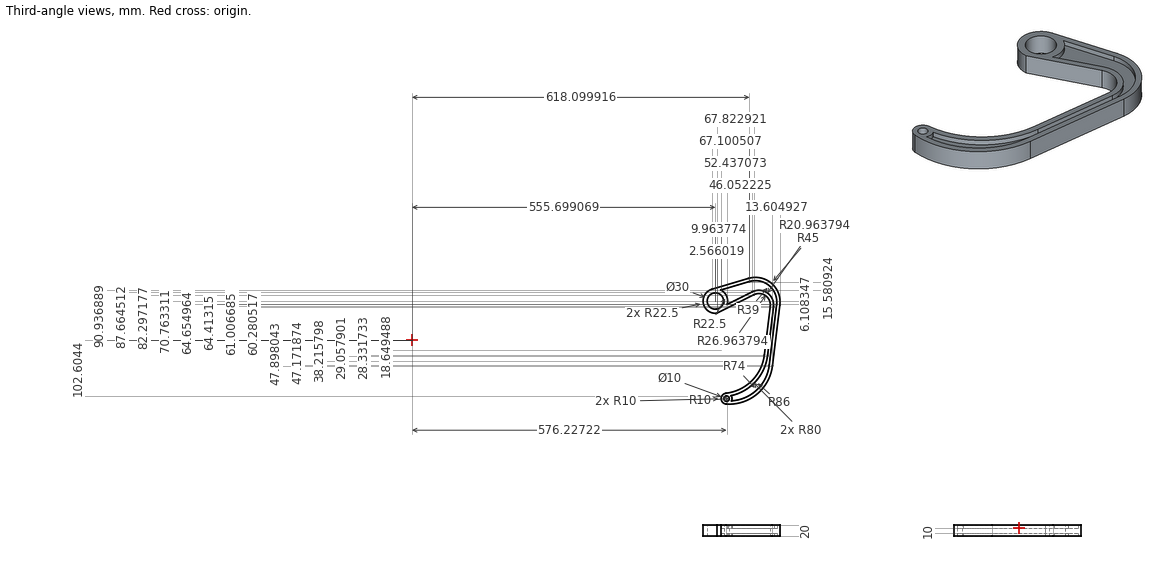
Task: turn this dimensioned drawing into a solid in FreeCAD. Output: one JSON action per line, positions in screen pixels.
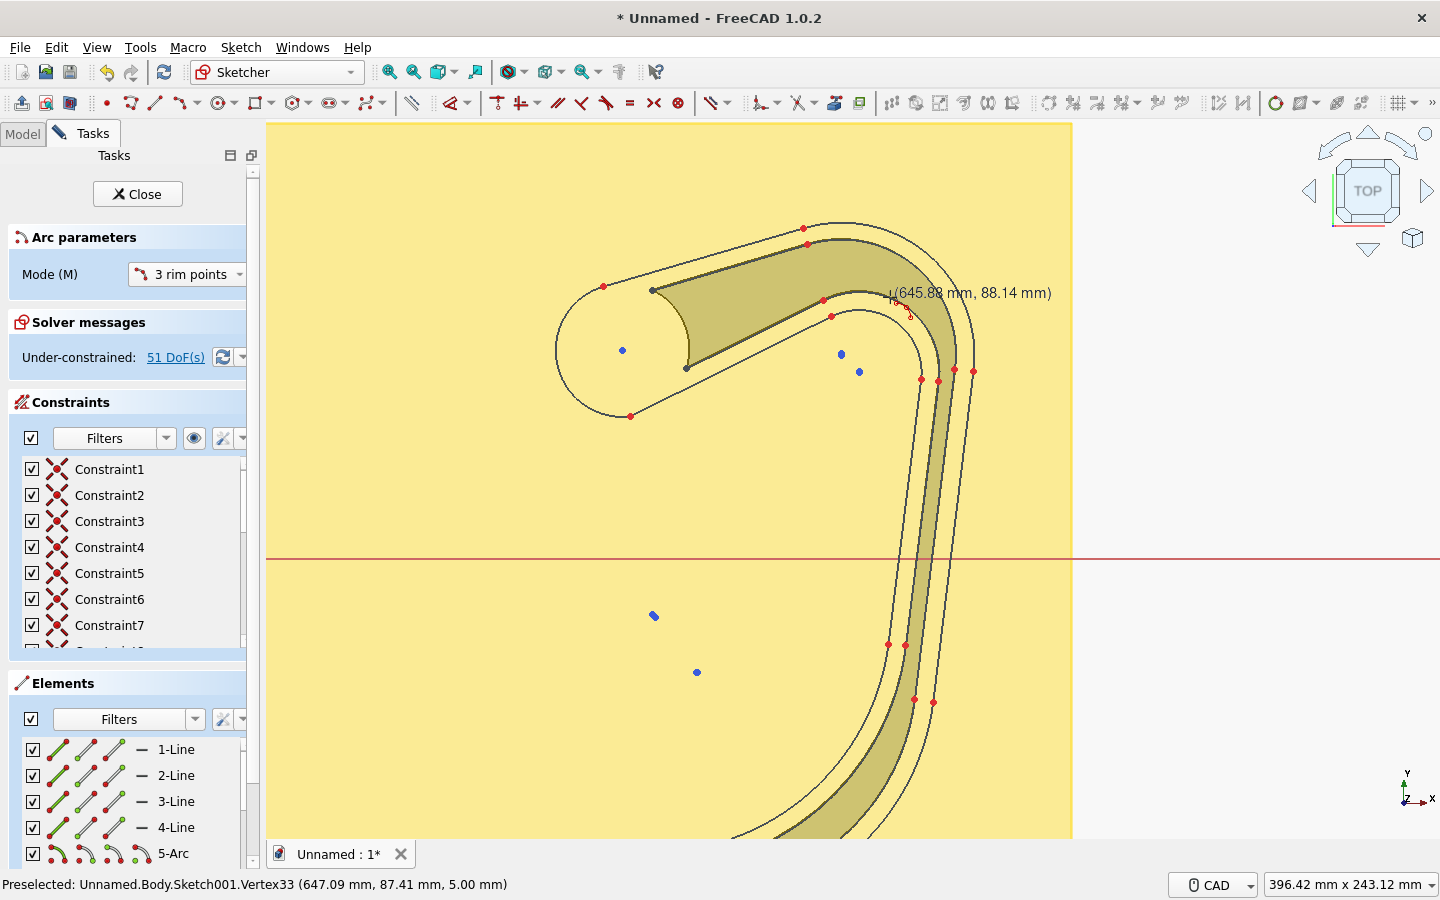
{"action": "left_click", "coordinate": [687, 369]}
{"action": "left_click", "coordinate": [653, 291]}
{"action": "left_click", "coordinate": [684, 322]}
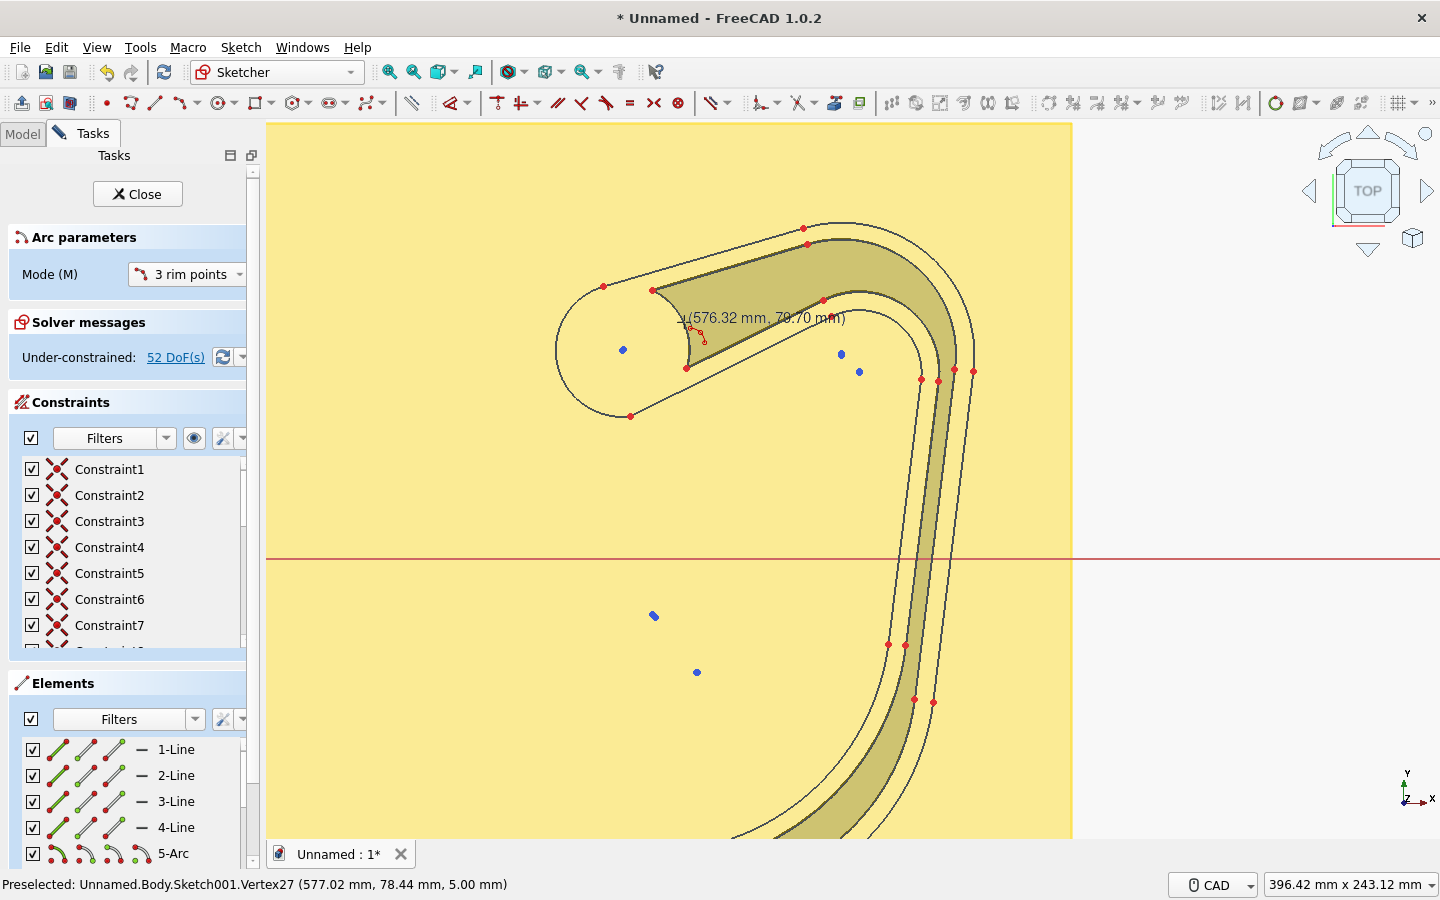
{"action": "left_click", "coordinate": [218, 104]}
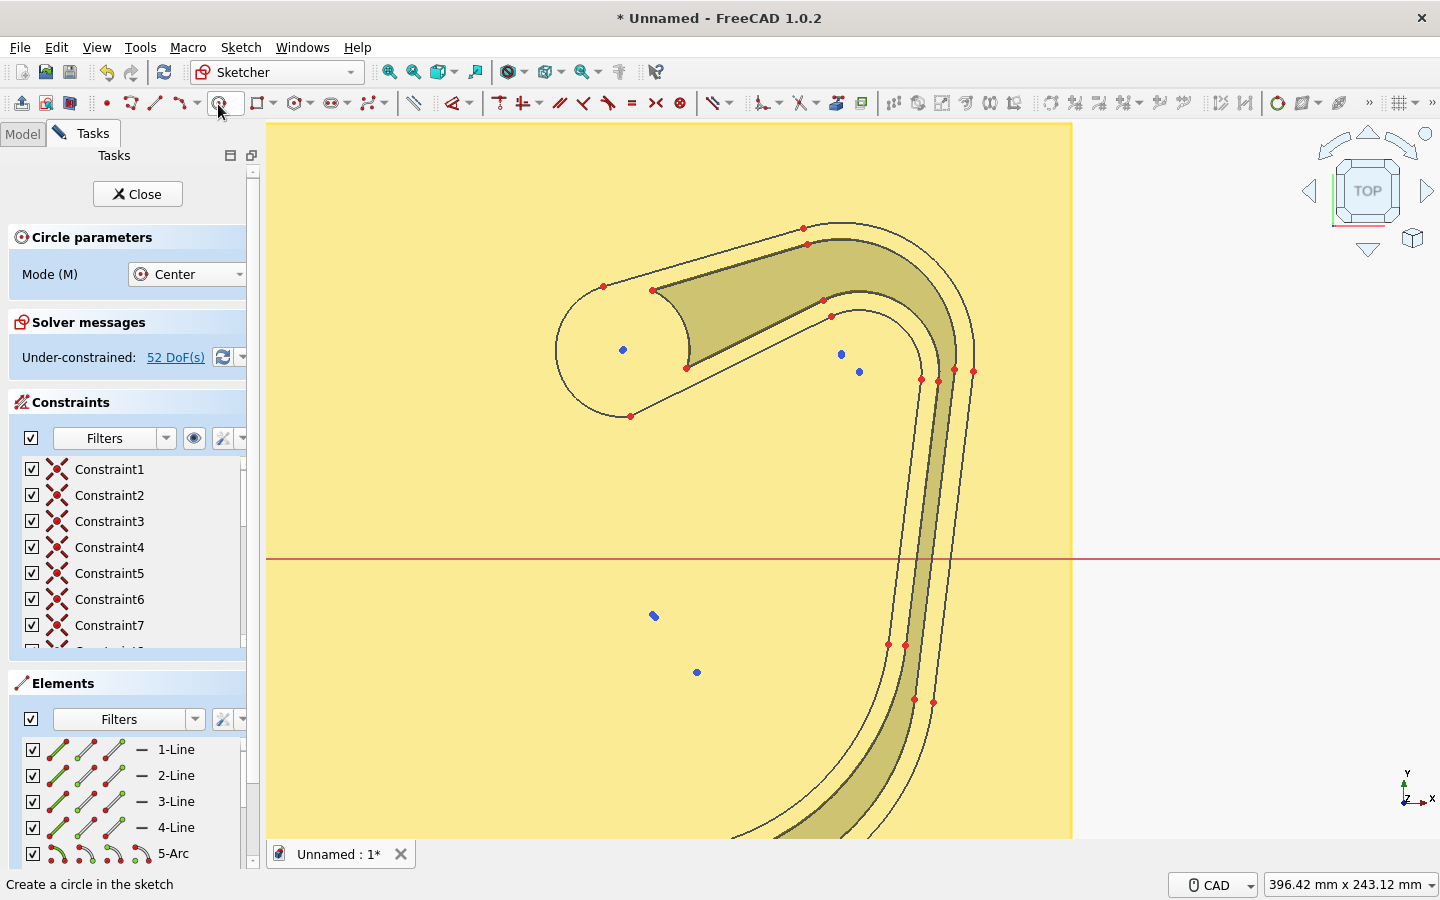
{"action": "scroll", "coordinate": [824, 299], "scroll_direction": "down", "scroll_amount": 2}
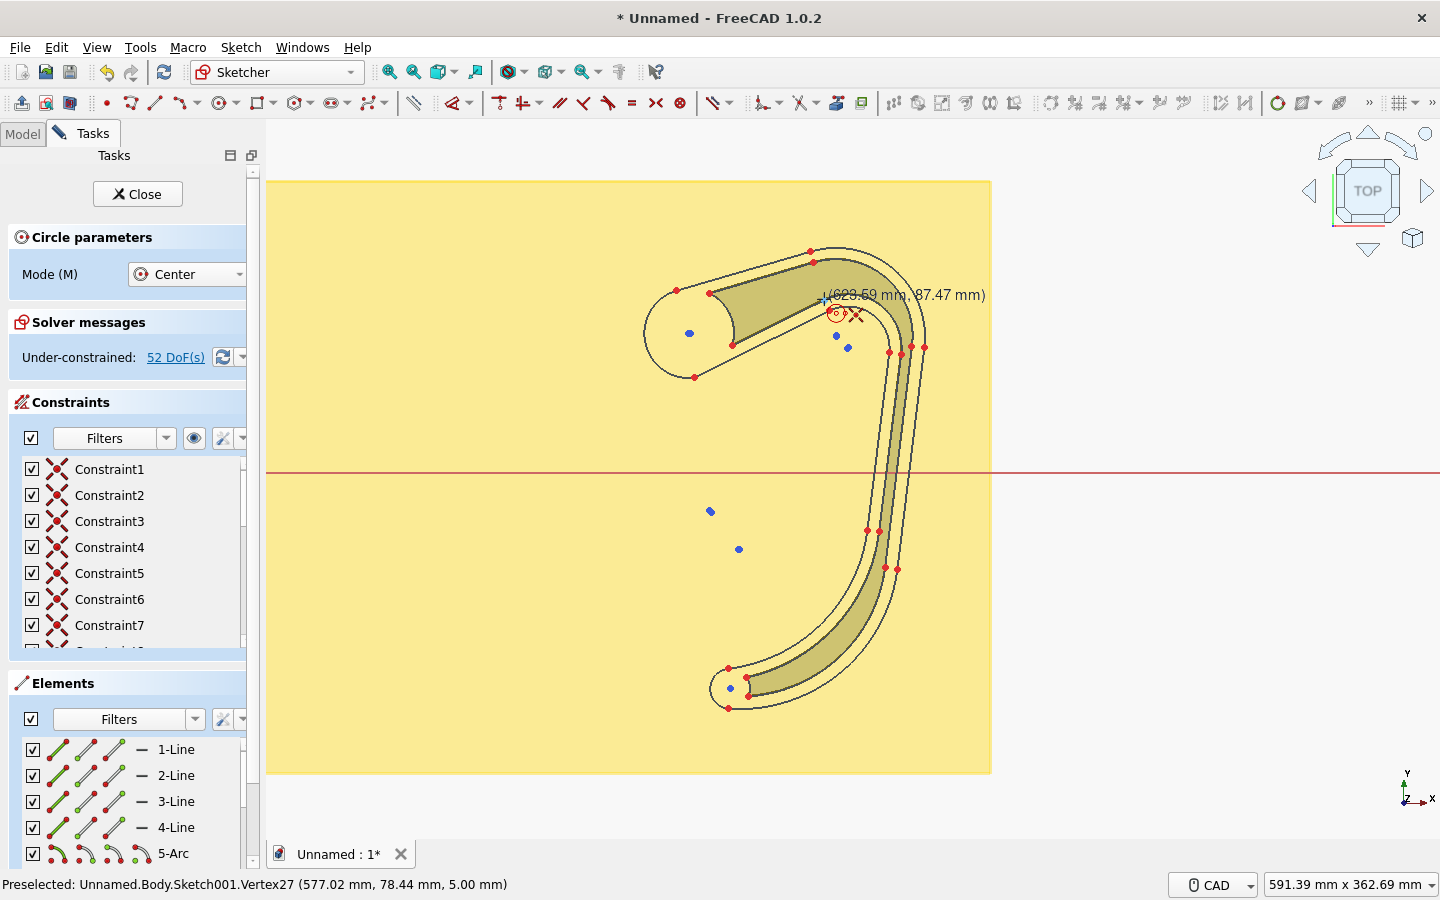
{"action": "scroll", "coordinate": [730, 688], "scroll_direction": "up", "scroll_amount": 5}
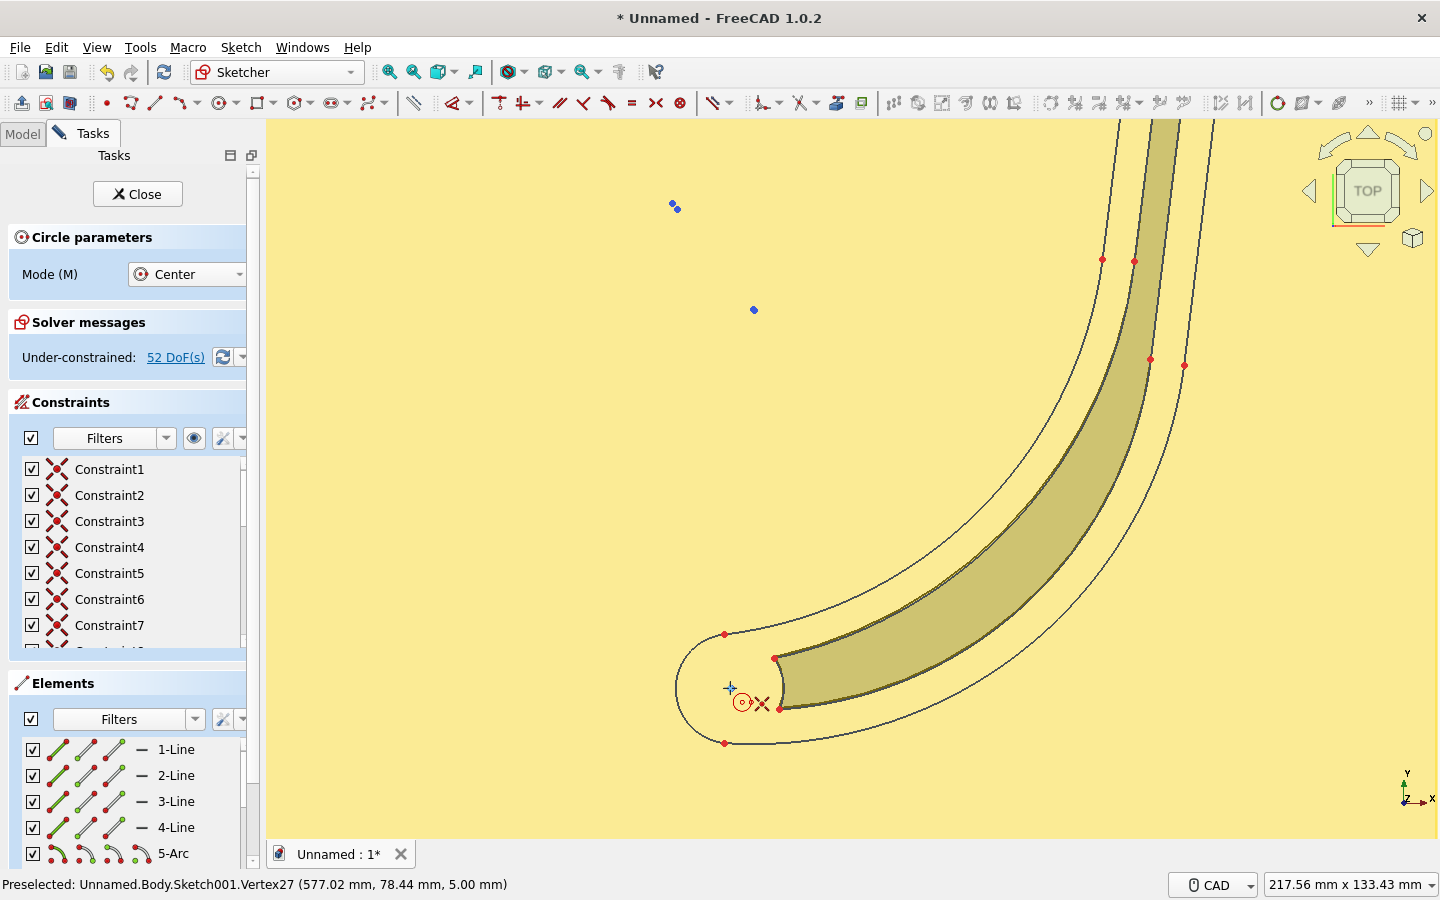
{"action": "left_click", "coordinate": [730, 686]}
{"action": "mouse_move", "coordinate": [749, 667]}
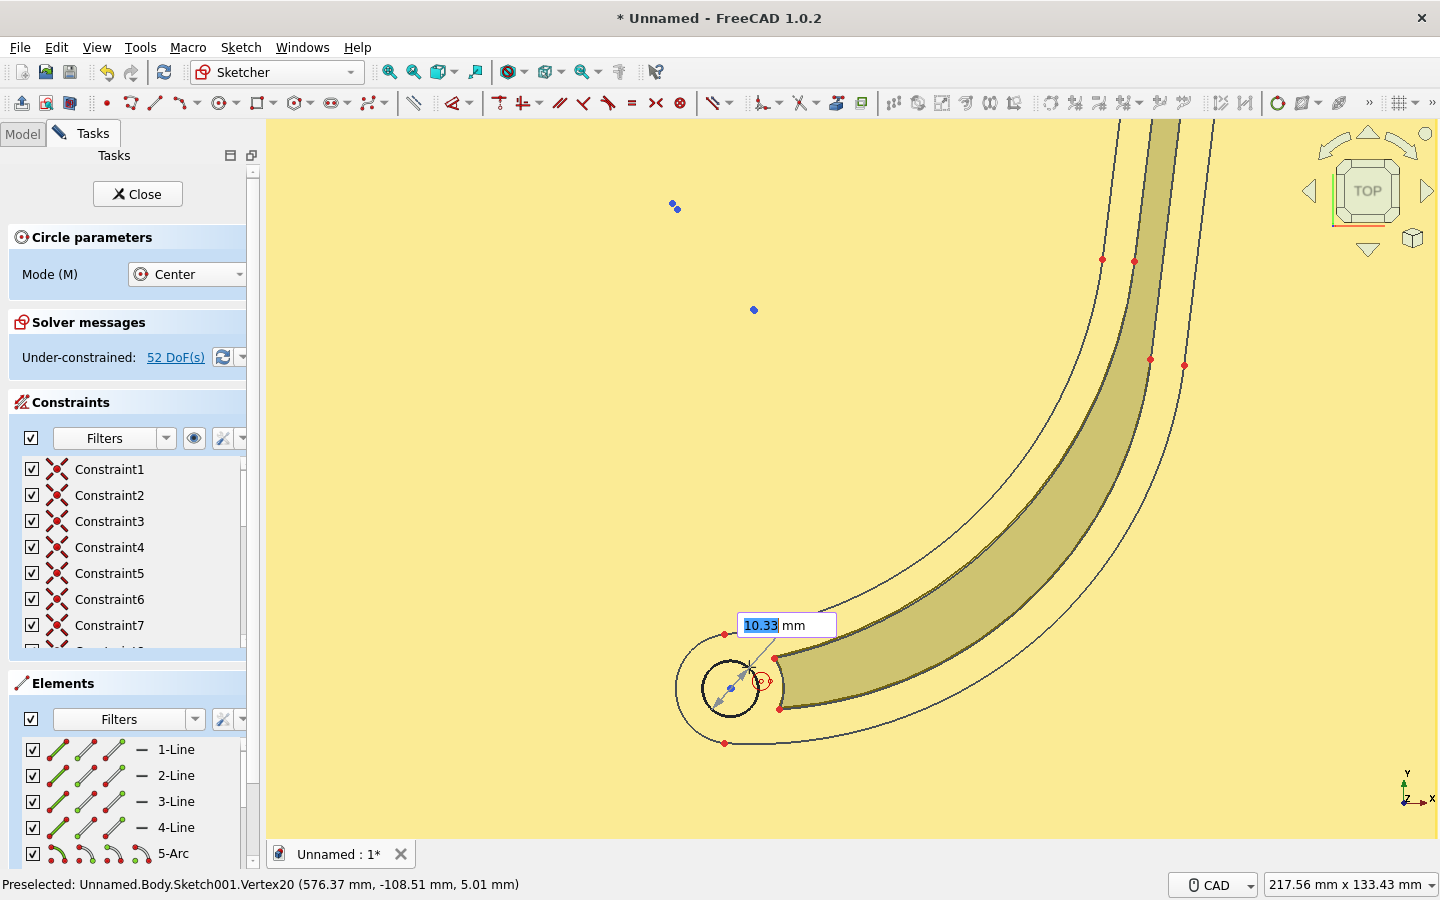
{"action": "type", "text": "10"}
{"action": "key", "text": "Return"}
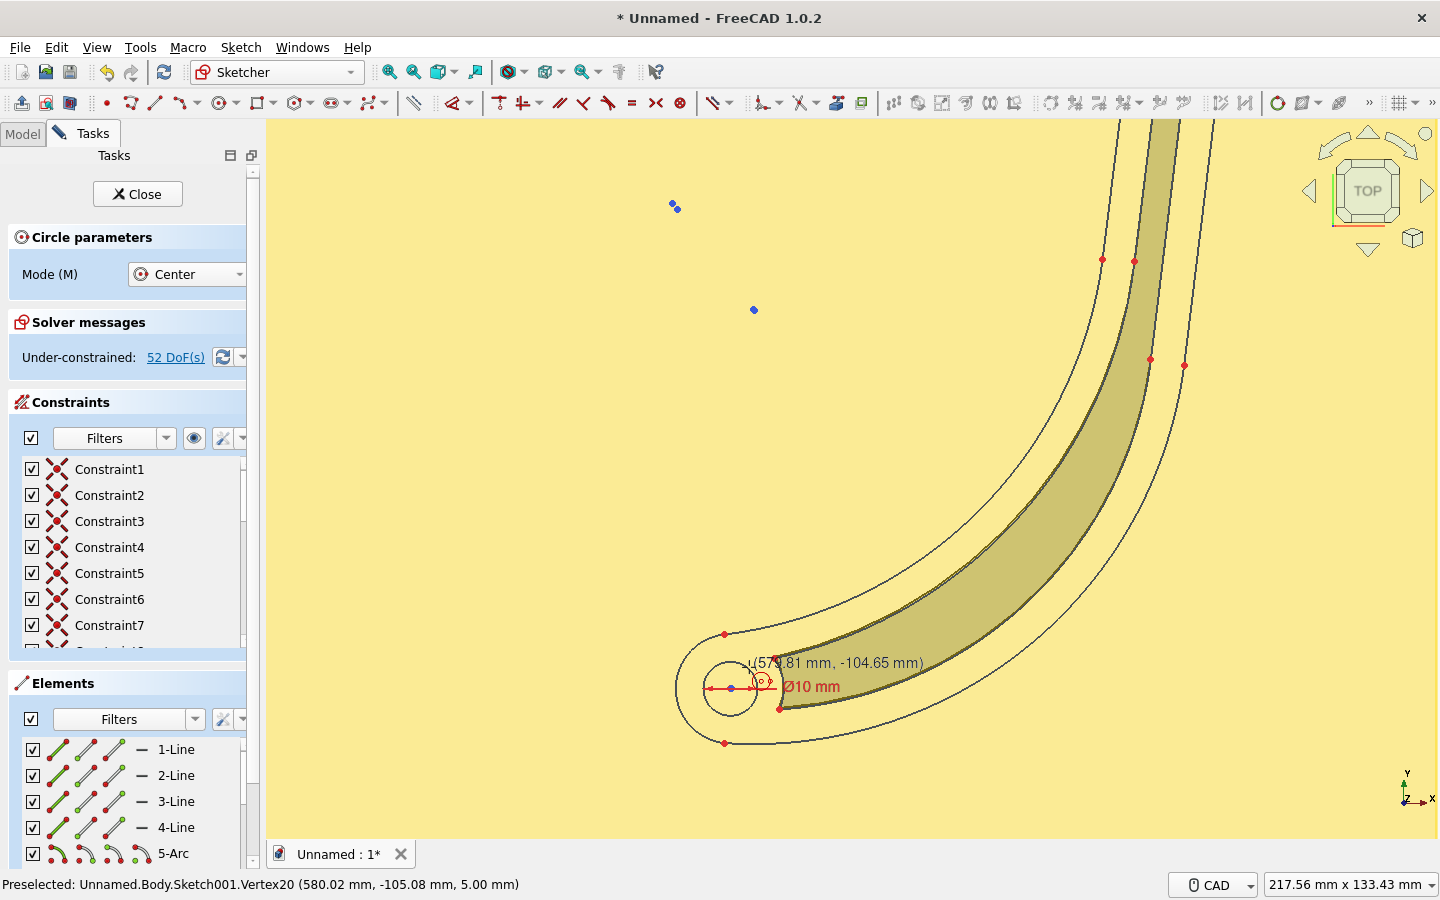
{"action": "scroll", "coordinate": [730, 689], "scroll_direction": "down", "scroll_amount": 5}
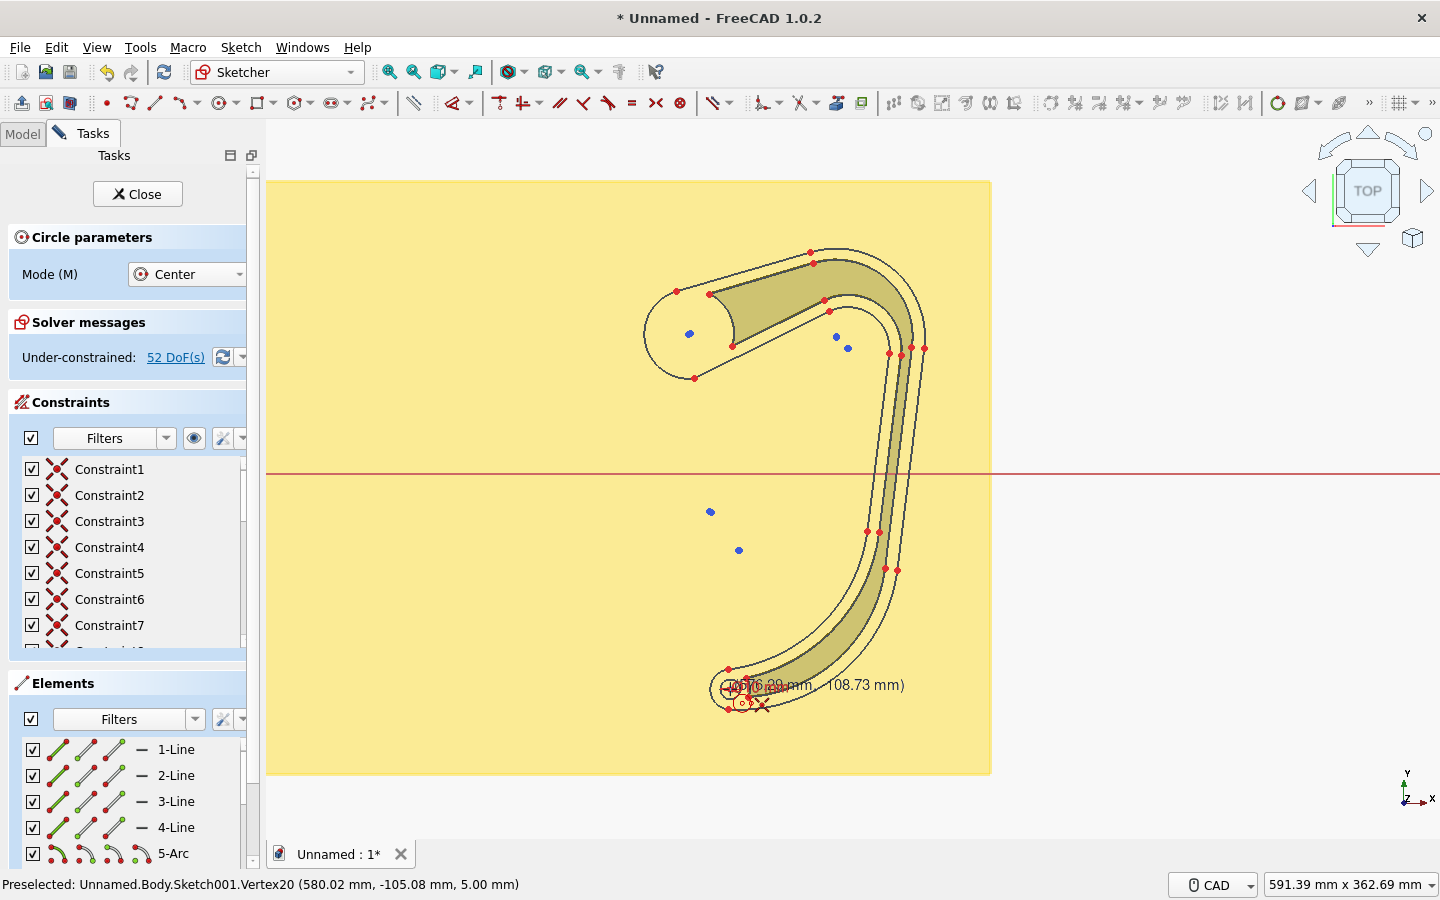
{"action": "left_click", "coordinate": [689, 334]}
{"action": "mouse_move", "coordinate": [710, 312]}